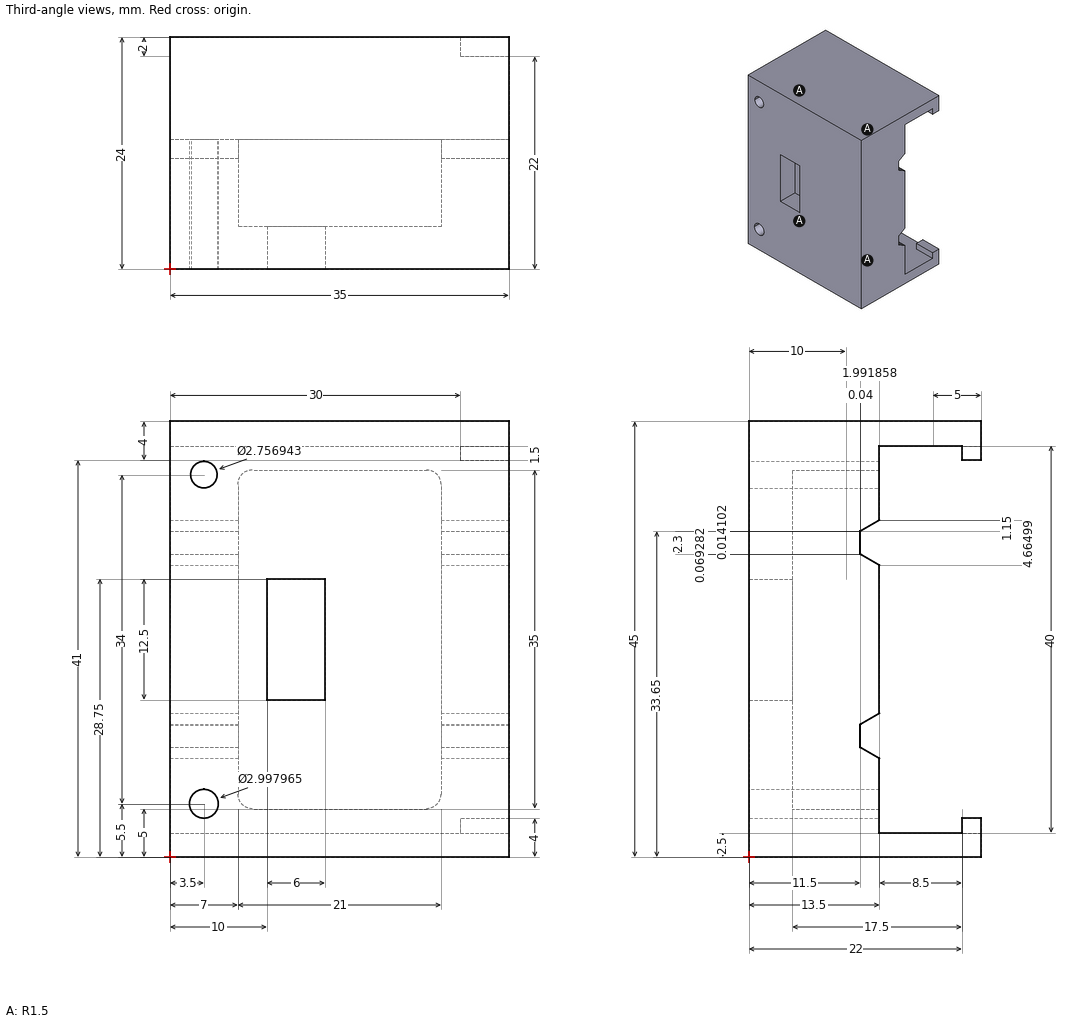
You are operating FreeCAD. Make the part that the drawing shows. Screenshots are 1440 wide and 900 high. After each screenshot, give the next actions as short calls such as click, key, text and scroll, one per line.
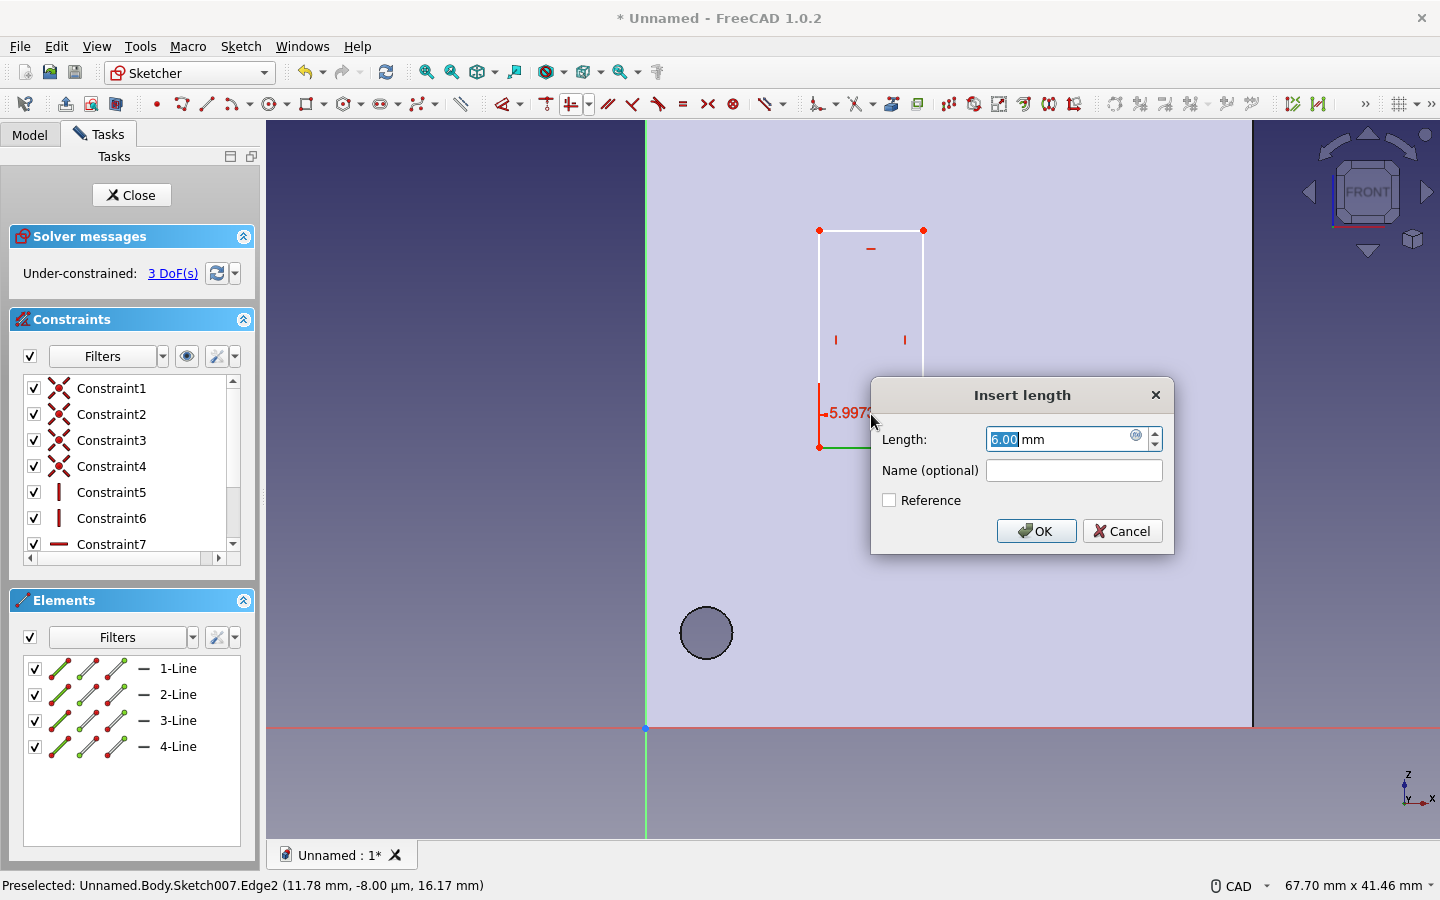
text(6)
key(Return)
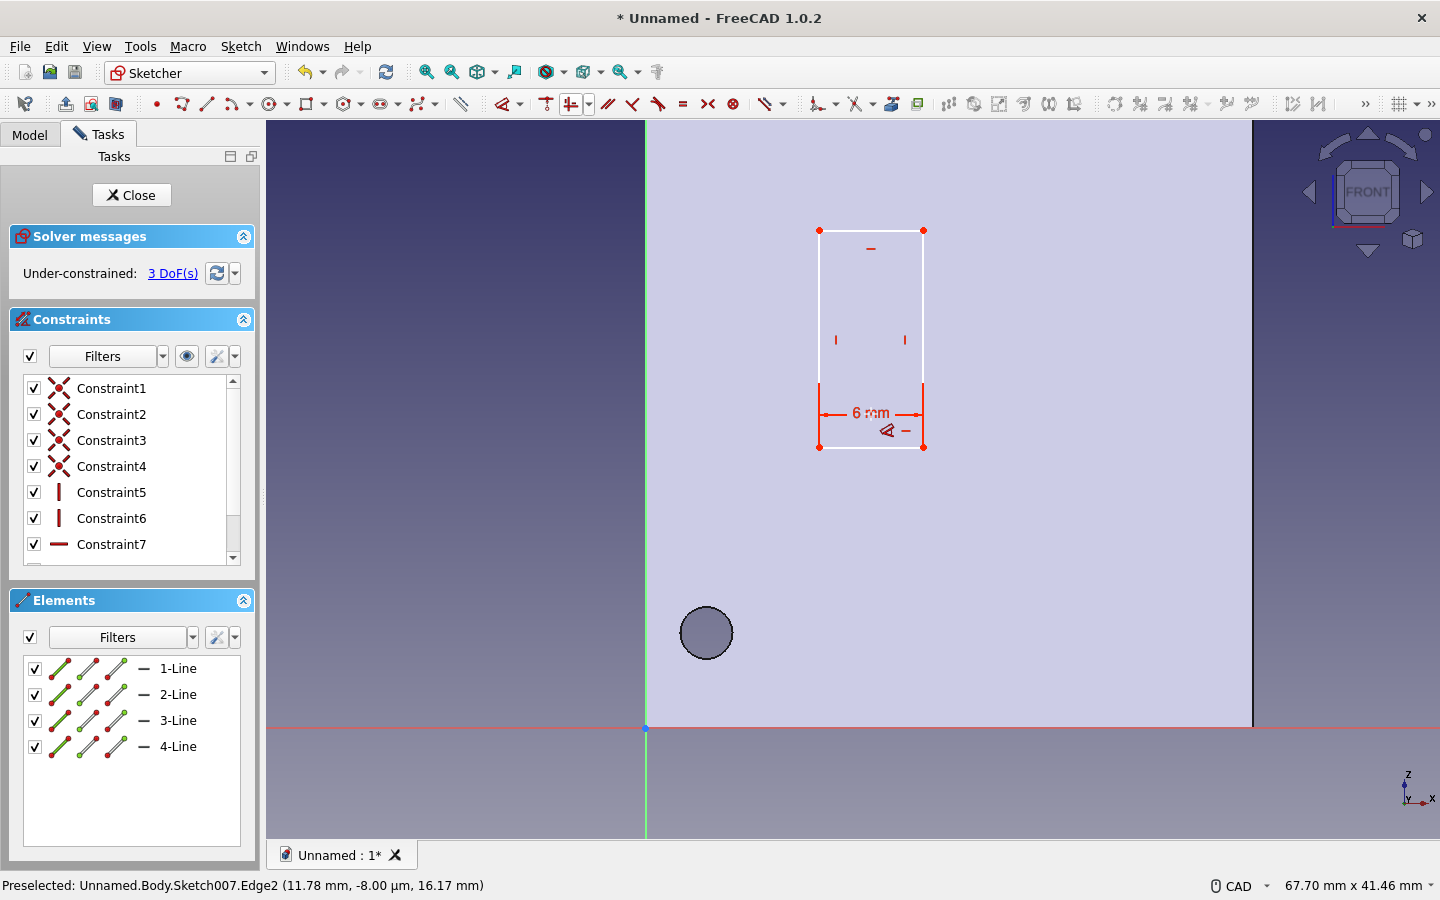
click(819, 231)
click(732, 762)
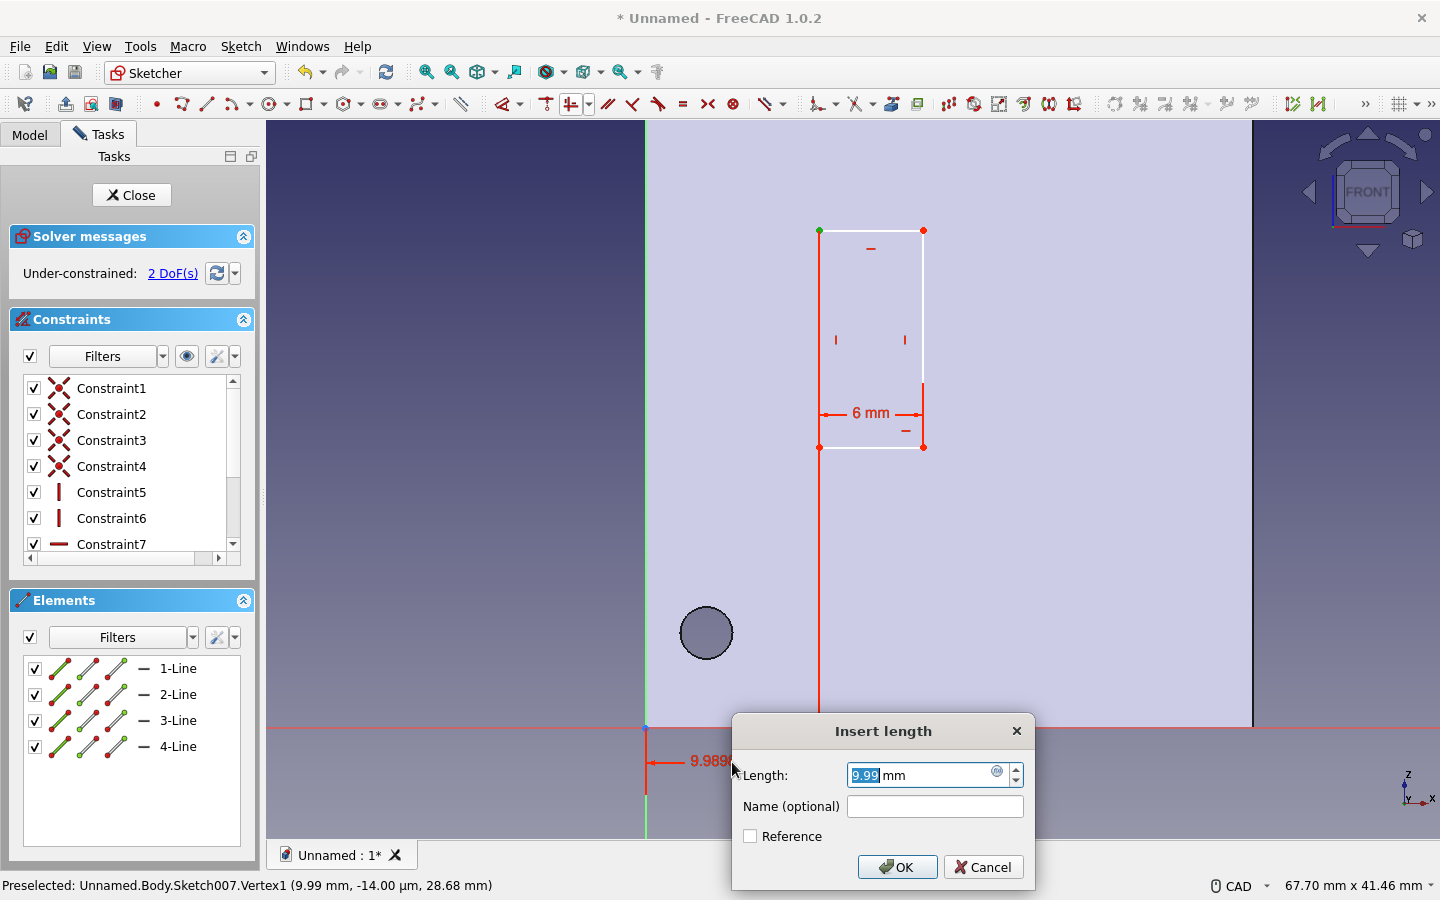
text(10)
key(Return)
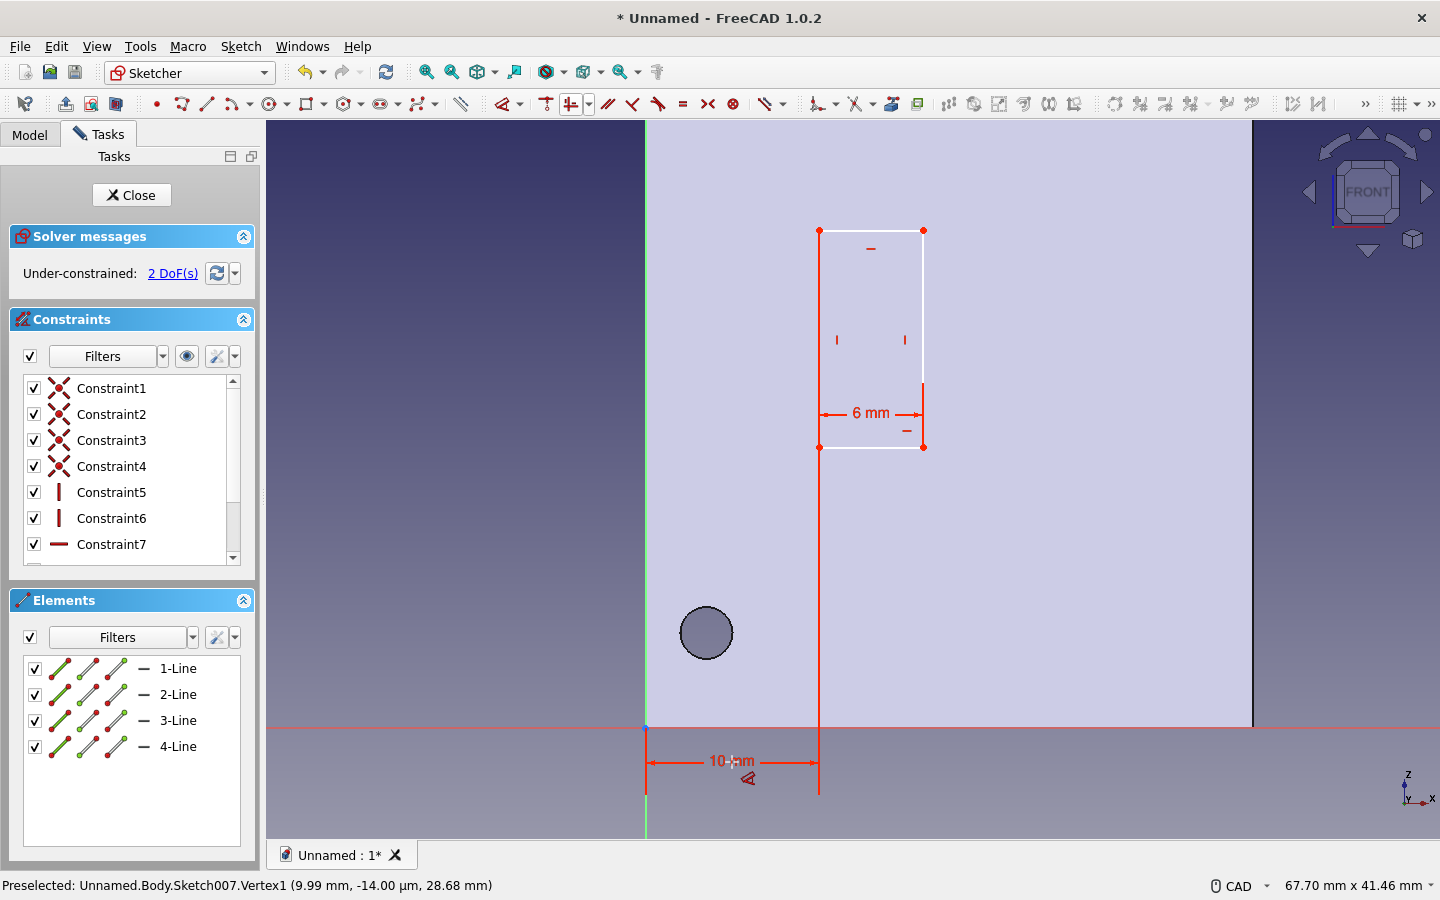
click(819, 296)
click(853, 340)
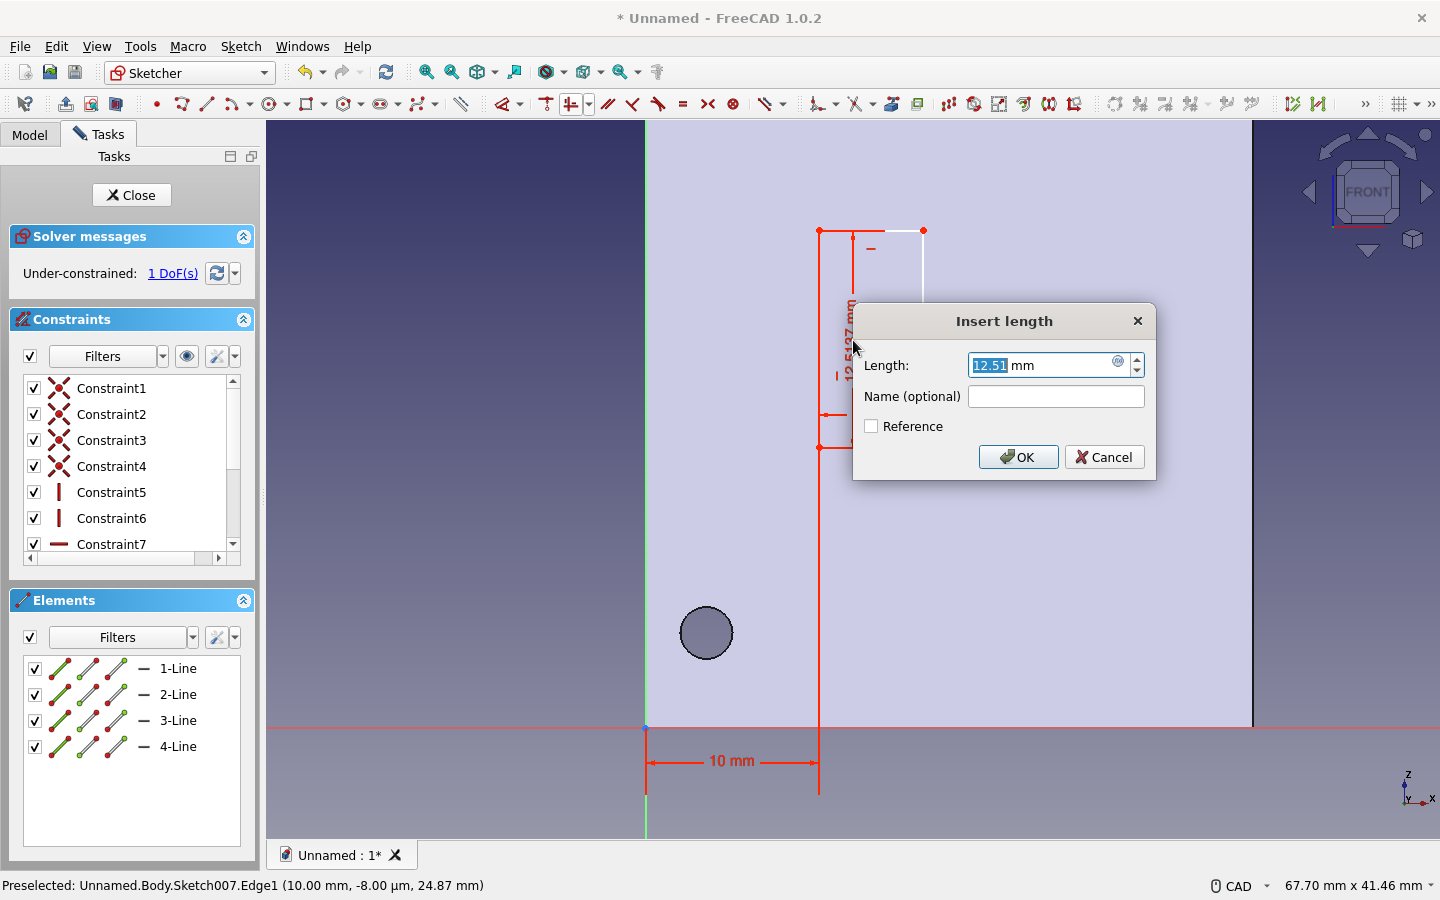
text(12.5)
key(Return)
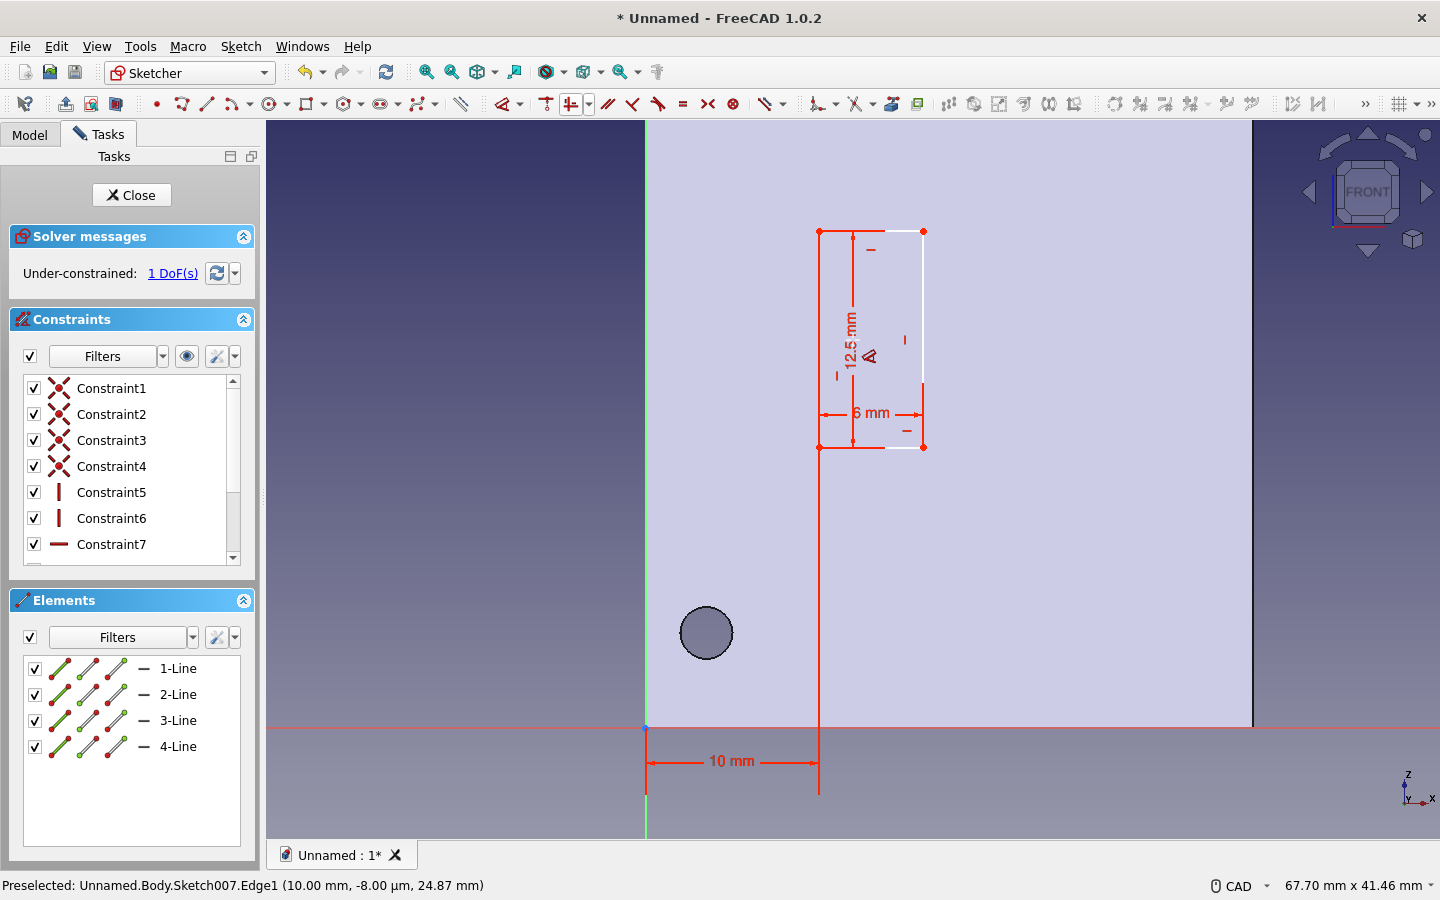
click(819, 231)
click(612, 480)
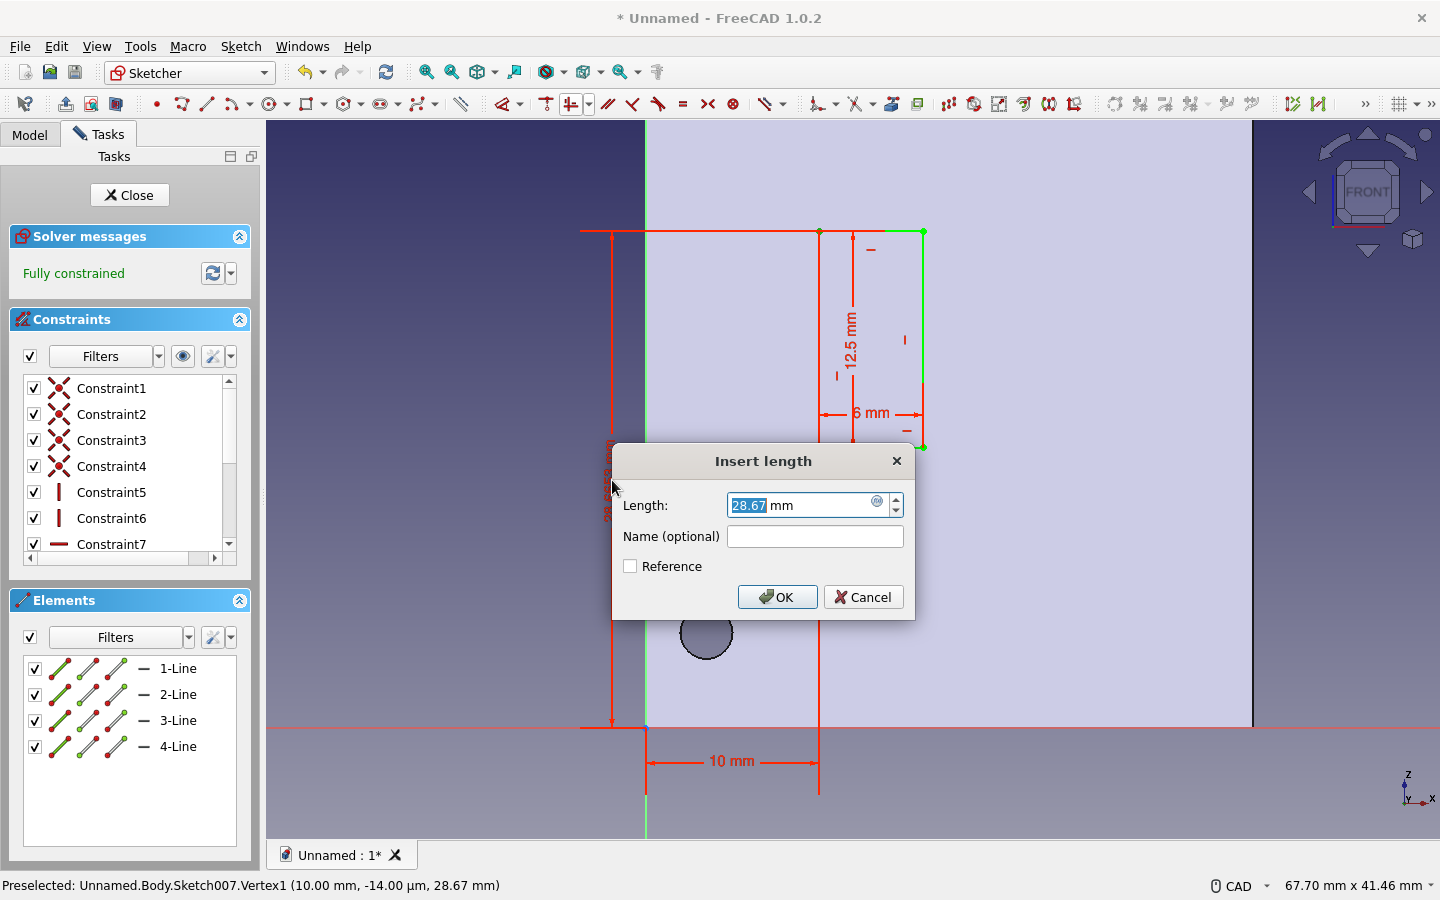
text(28.75)
key(Return)
key(Escape)